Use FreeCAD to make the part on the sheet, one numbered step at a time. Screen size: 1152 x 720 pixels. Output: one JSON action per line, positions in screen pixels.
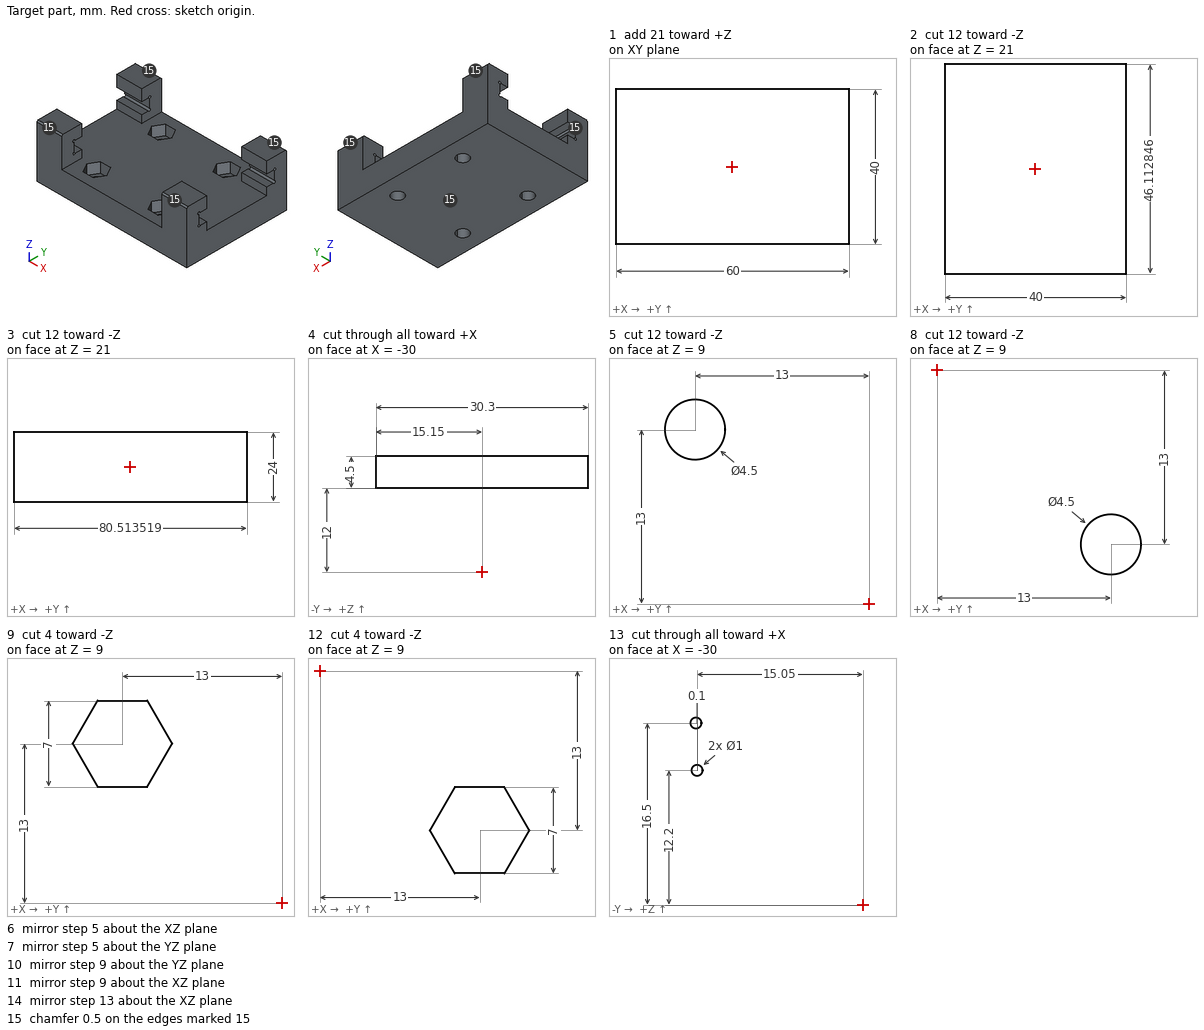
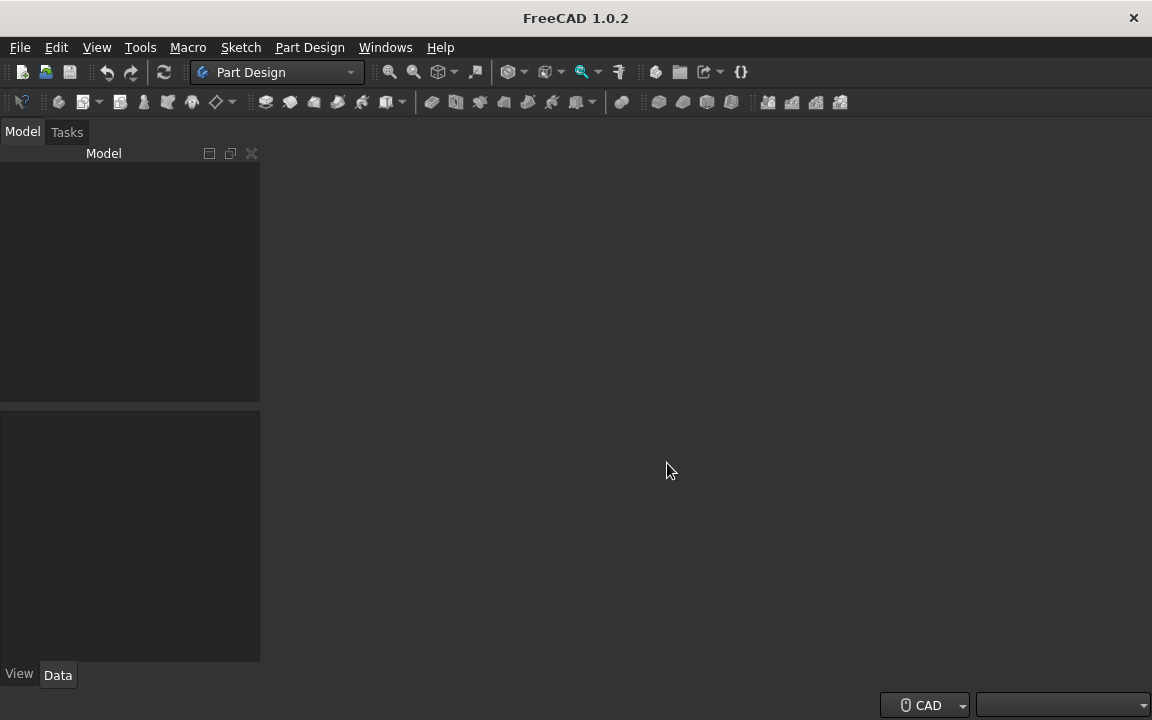
{"action": "left_click", "coordinate": [22, 72]}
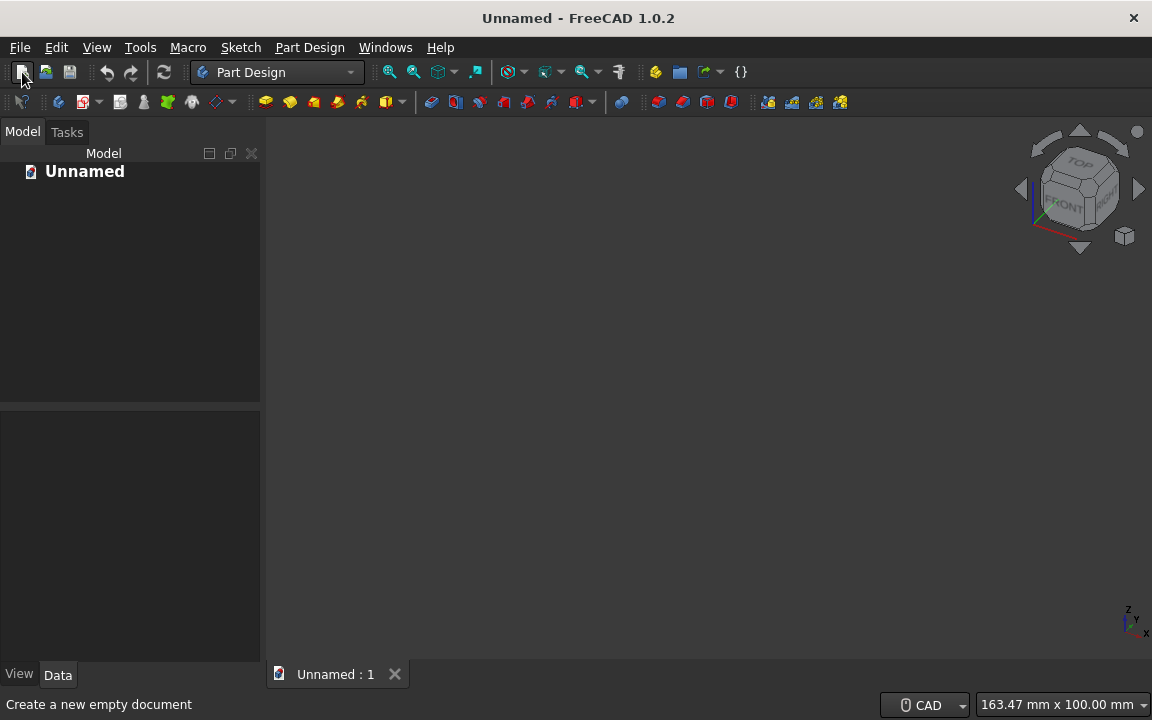
{"action": "left_click", "coordinate": [84, 102]}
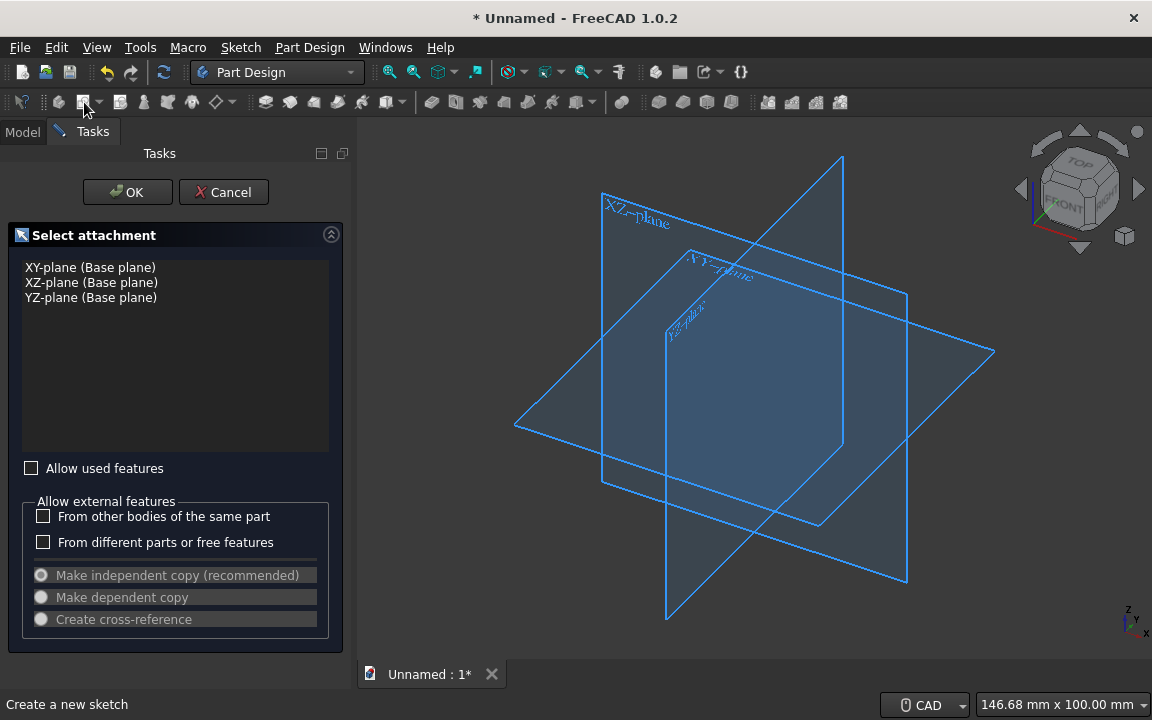
{"action": "left_click", "coordinate": [82, 268]}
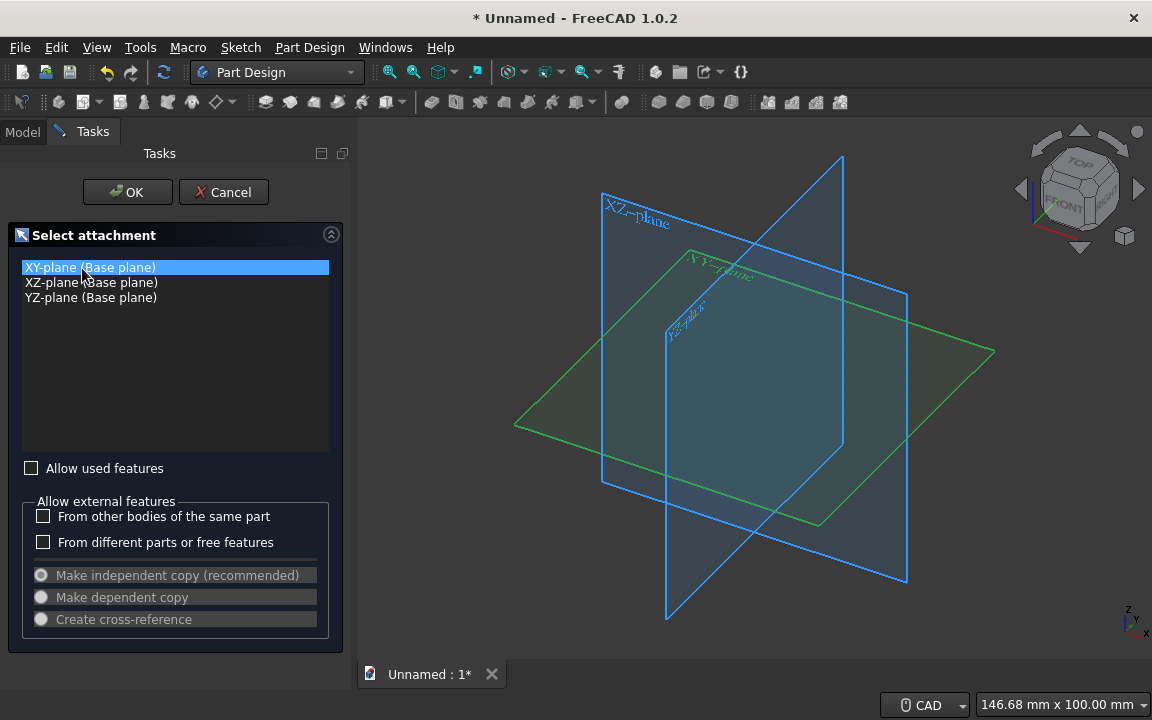
{"action": "left_click", "coordinate": [128, 192]}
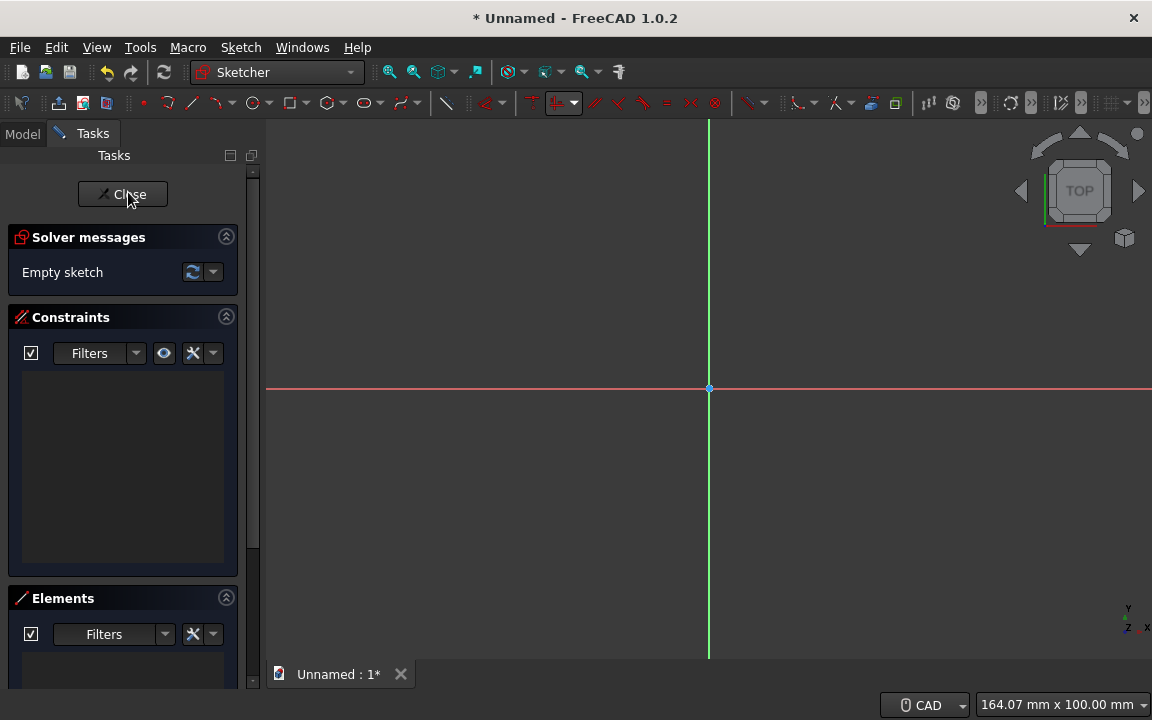
{"action": "scroll", "coordinate": [848, 389], "scroll_direction": "up", "scroll_amount": 2}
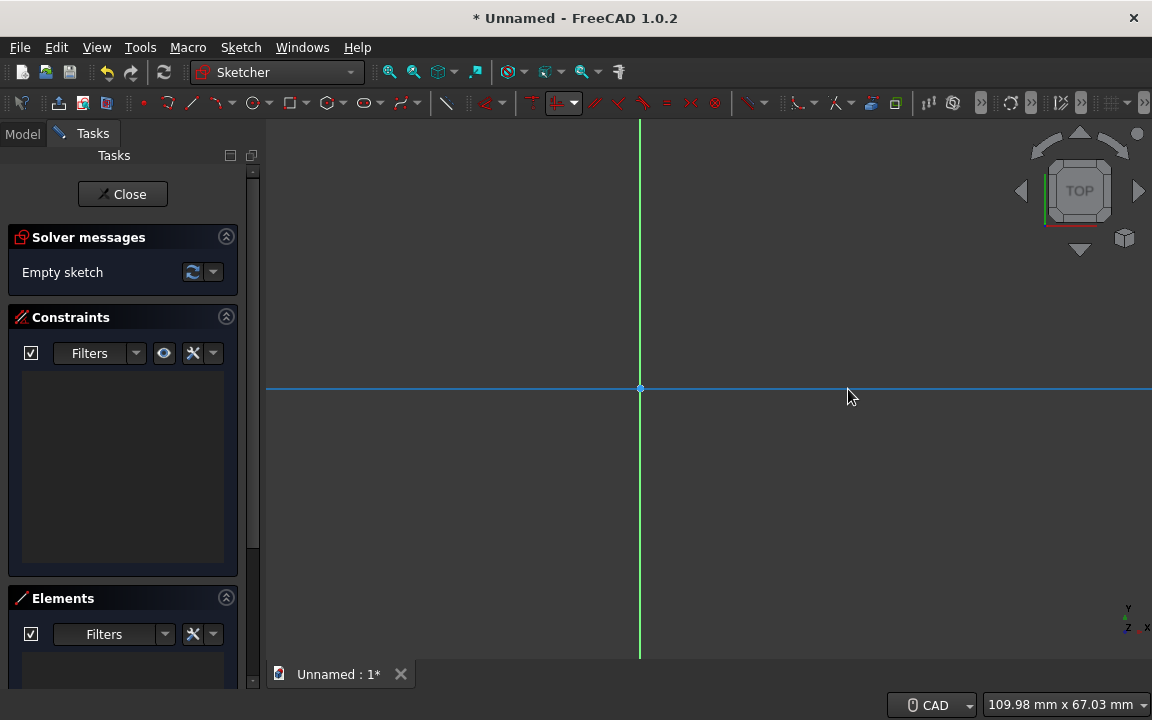
{"action": "left_click", "coordinate": [308, 104]}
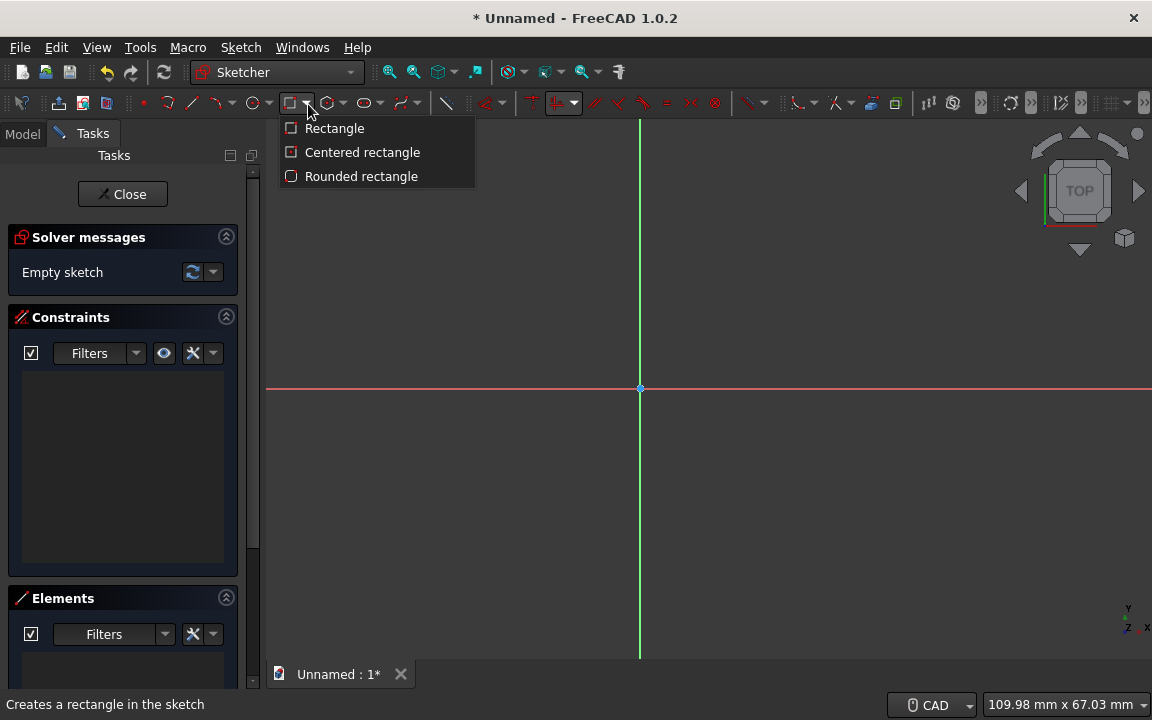
{"action": "left_click", "coordinate": [378, 152]}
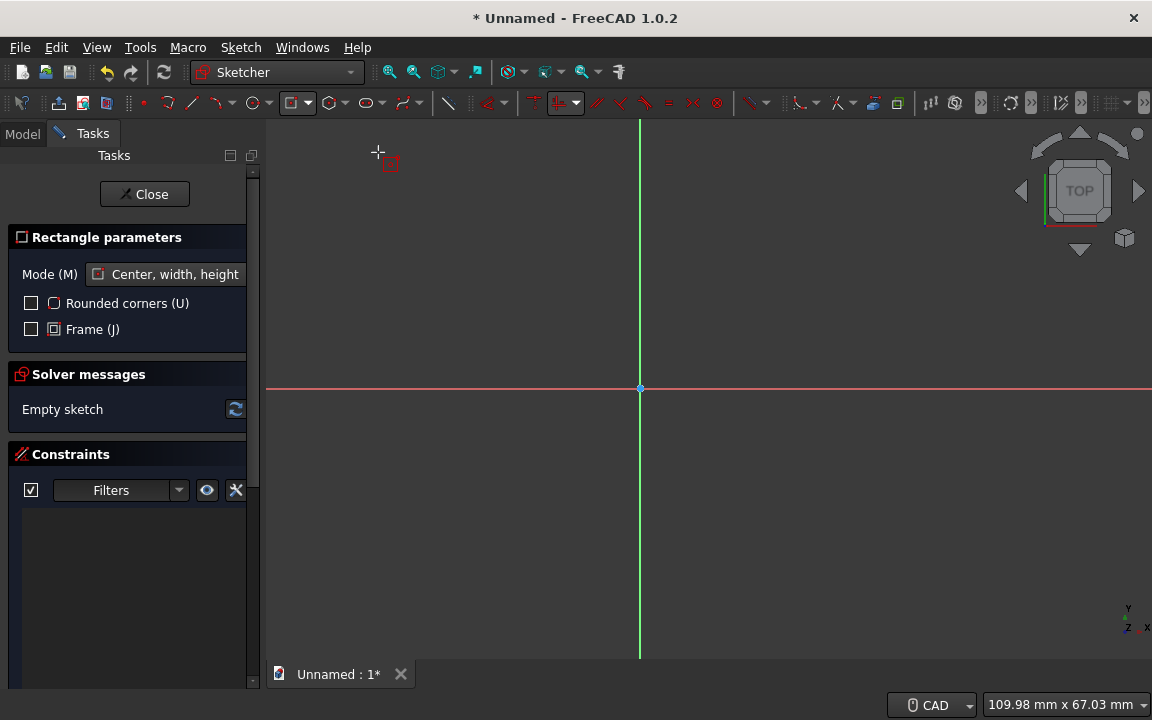
{"action": "left_click", "coordinate": [640, 389]}
{"action": "left_click", "coordinate": [882, 228]}
{"action": "key", "text": "Escape"}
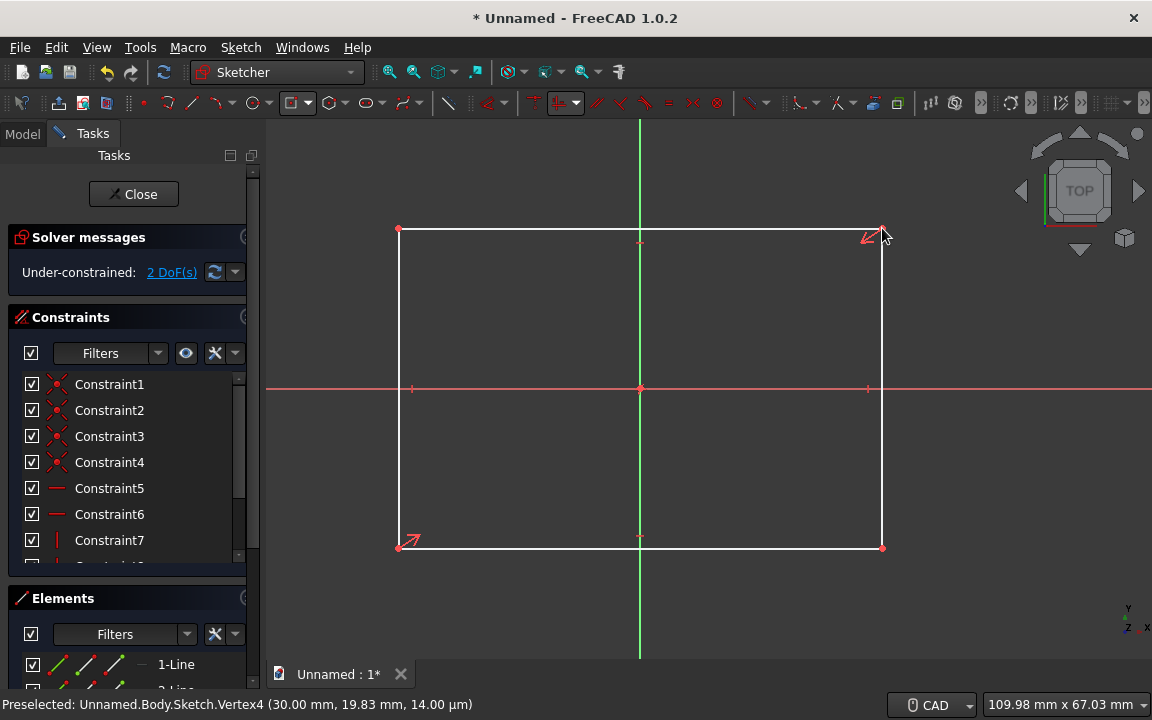
{"action": "left_click", "coordinate": [544, 549]}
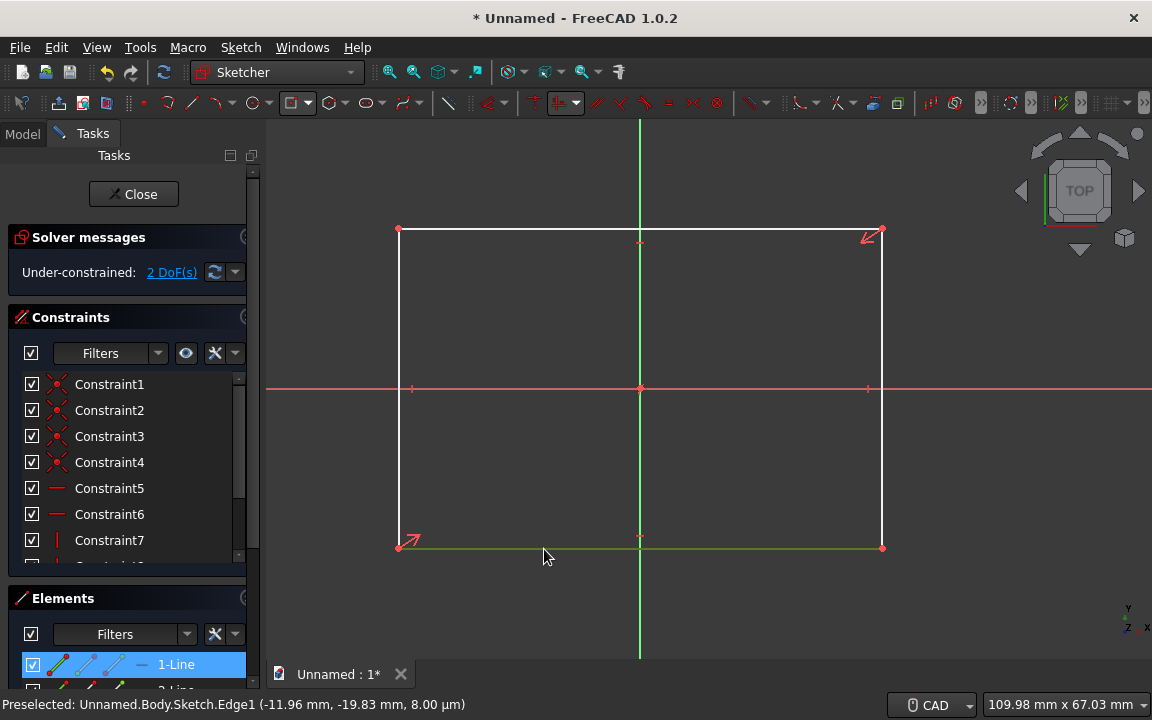
{"action": "left_click", "coordinate": [506, 104]}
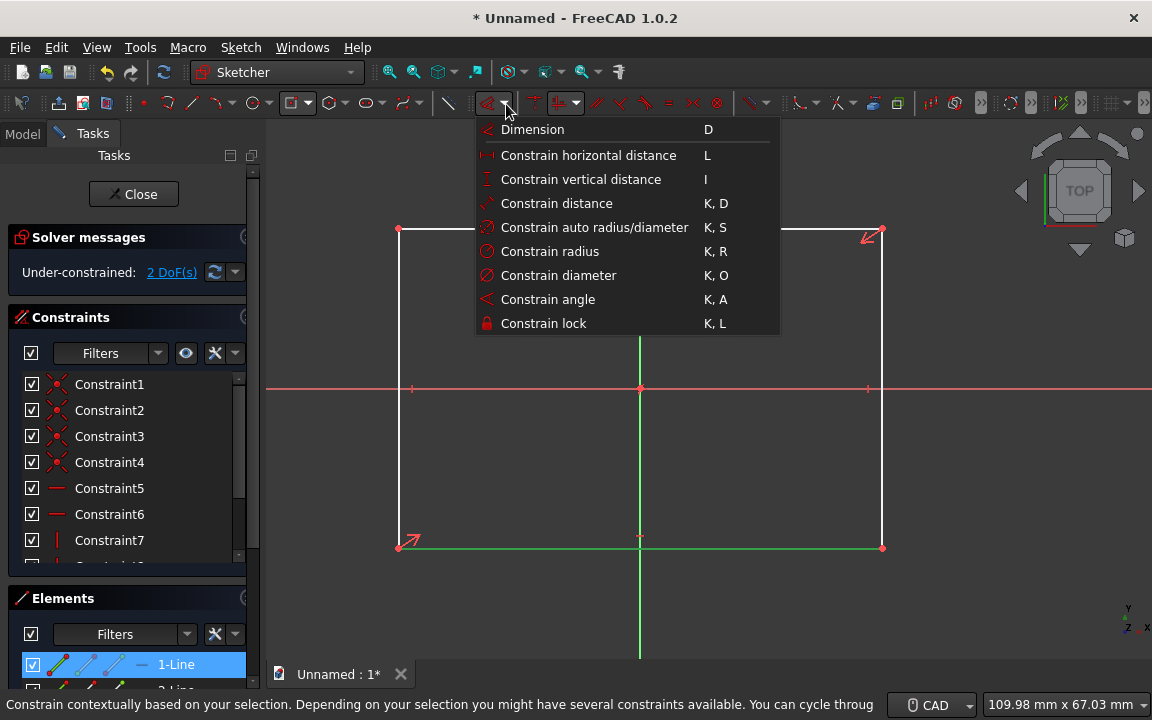
{"action": "left_click", "coordinate": [628, 155]}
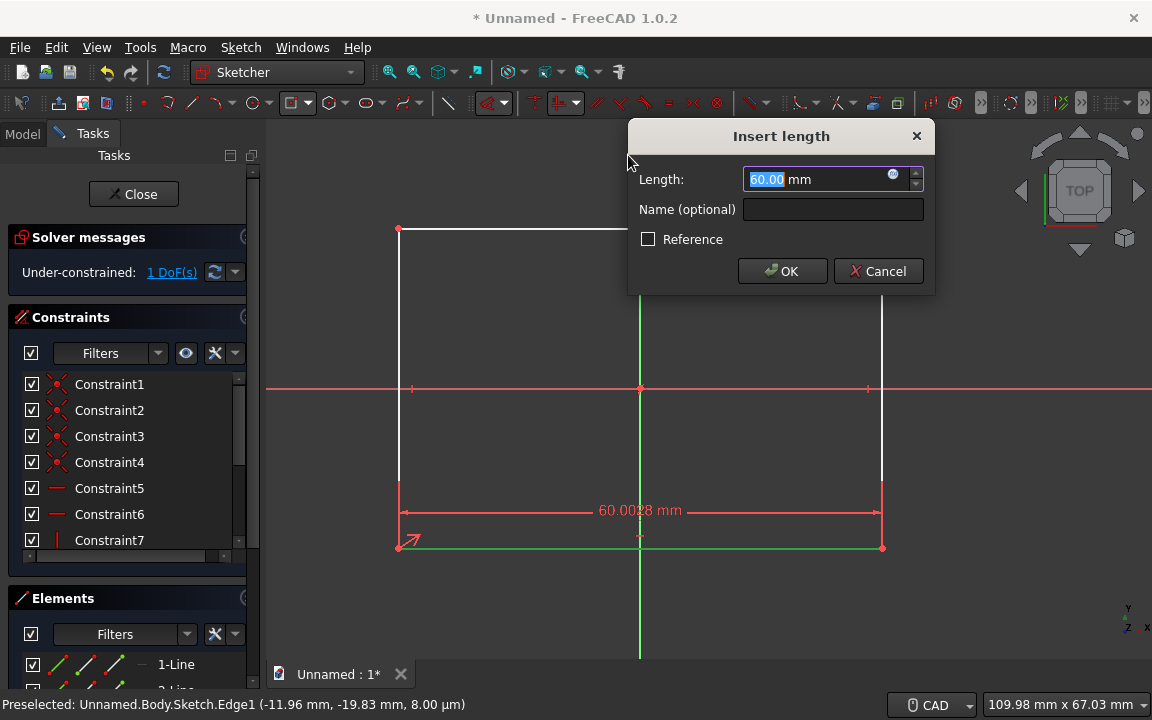
{"action": "type", "text": "60"}
{"action": "key", "text": "Return"}